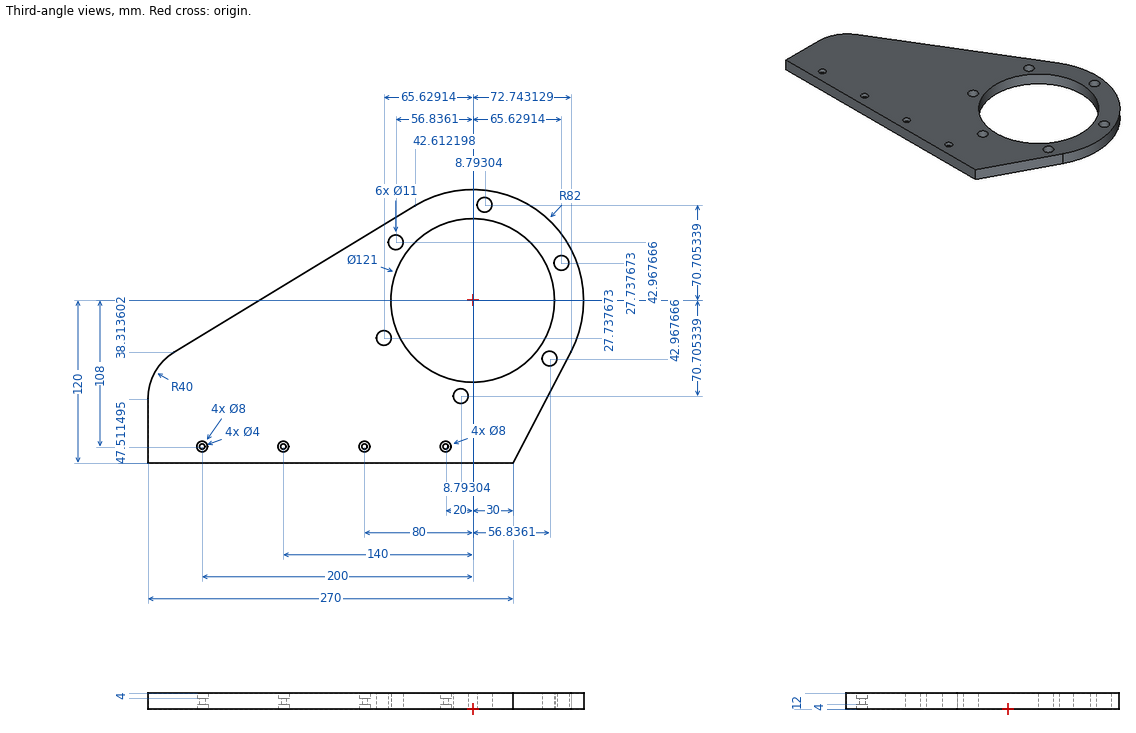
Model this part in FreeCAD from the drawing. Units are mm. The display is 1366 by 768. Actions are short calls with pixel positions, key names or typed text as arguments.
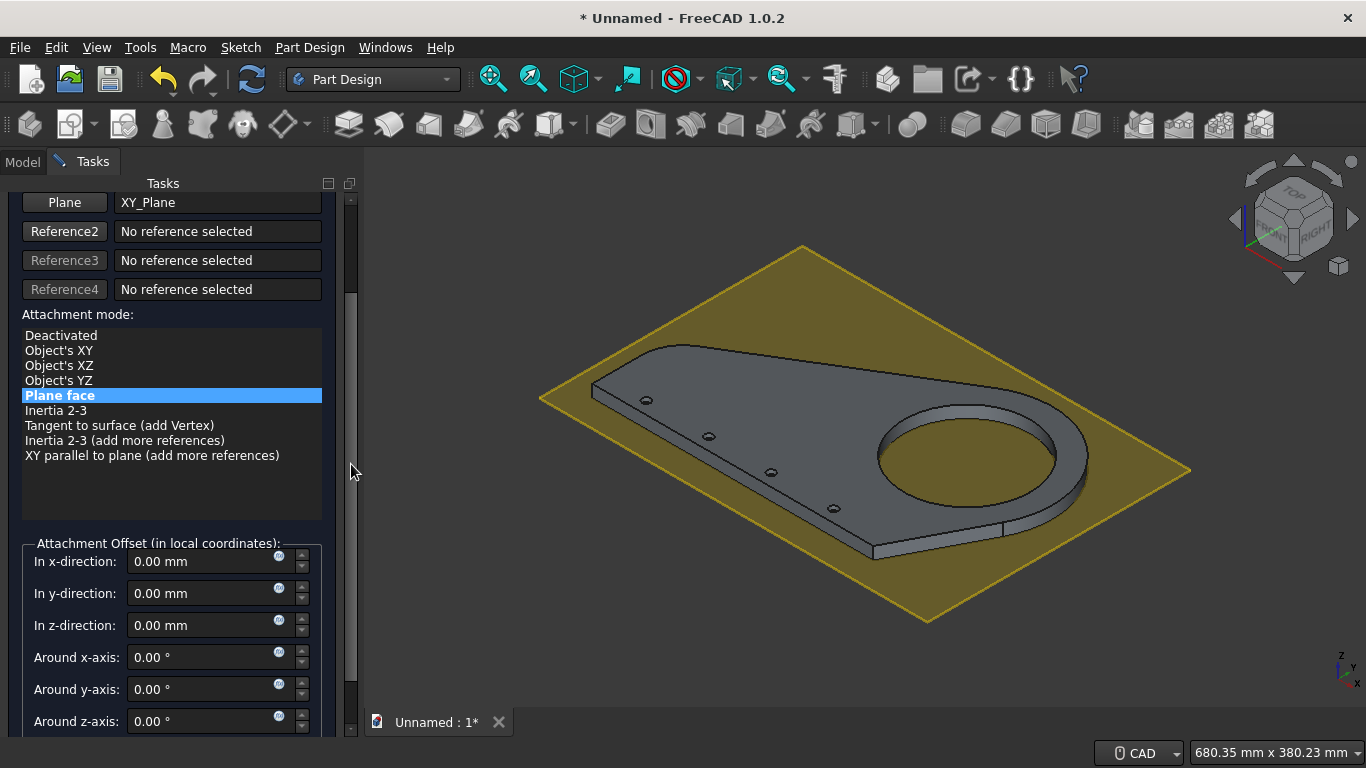
triple_click(210, 625)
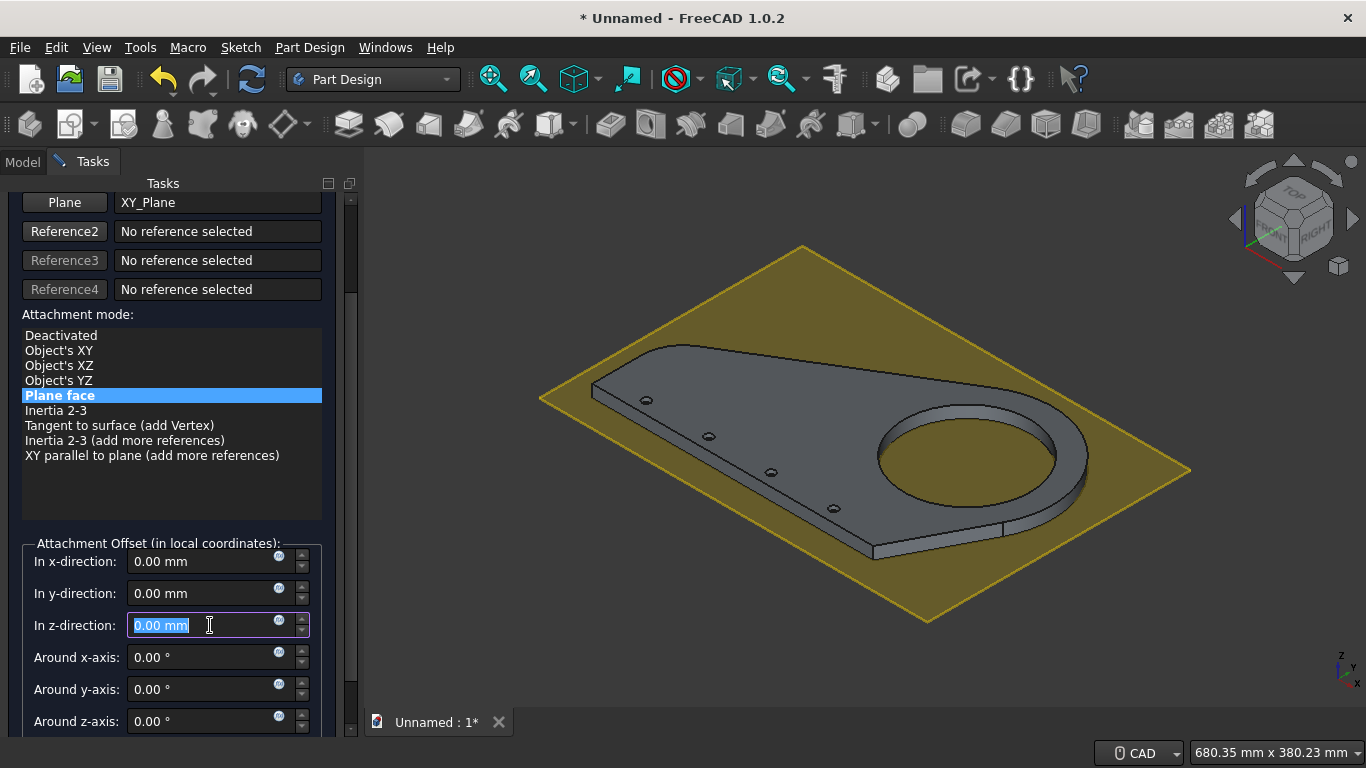
text(4)
key(Tab)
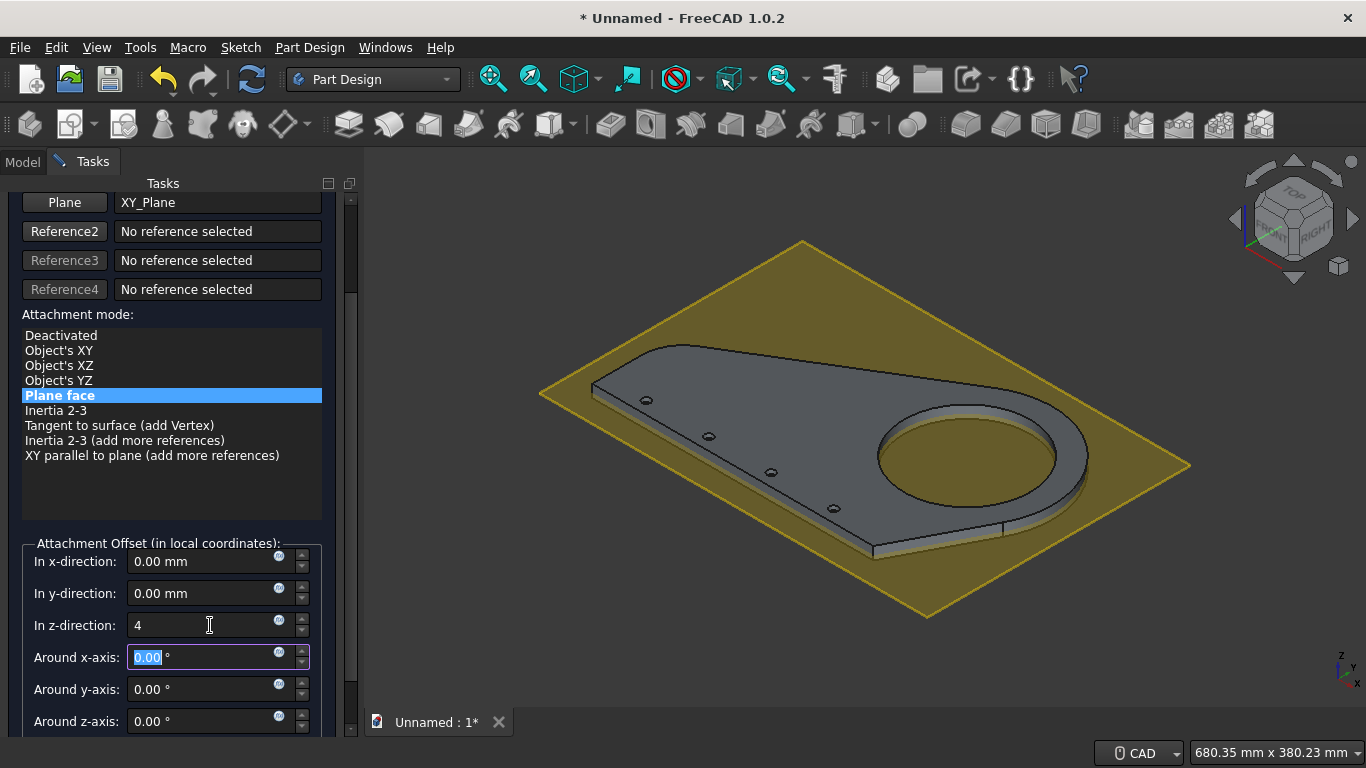
scroll(351, 464, up, 3)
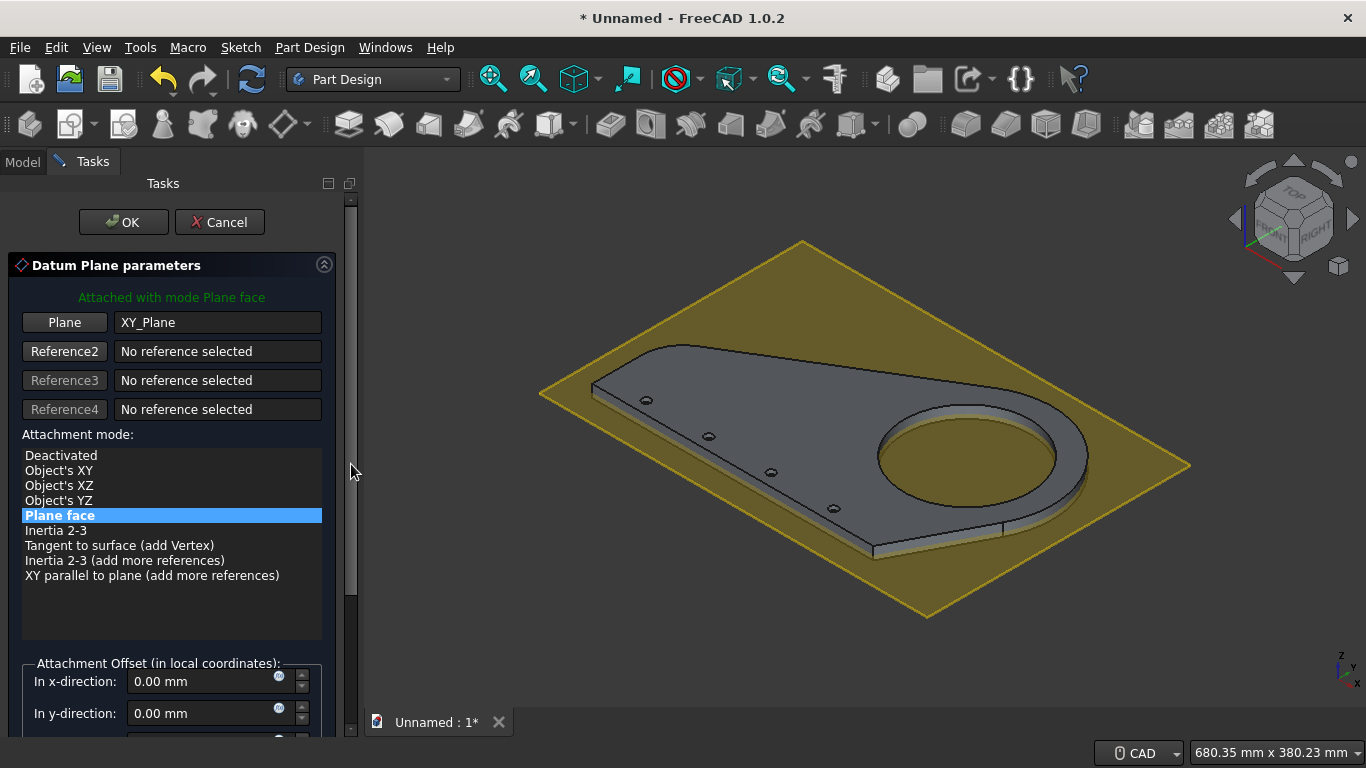
click(124, 222)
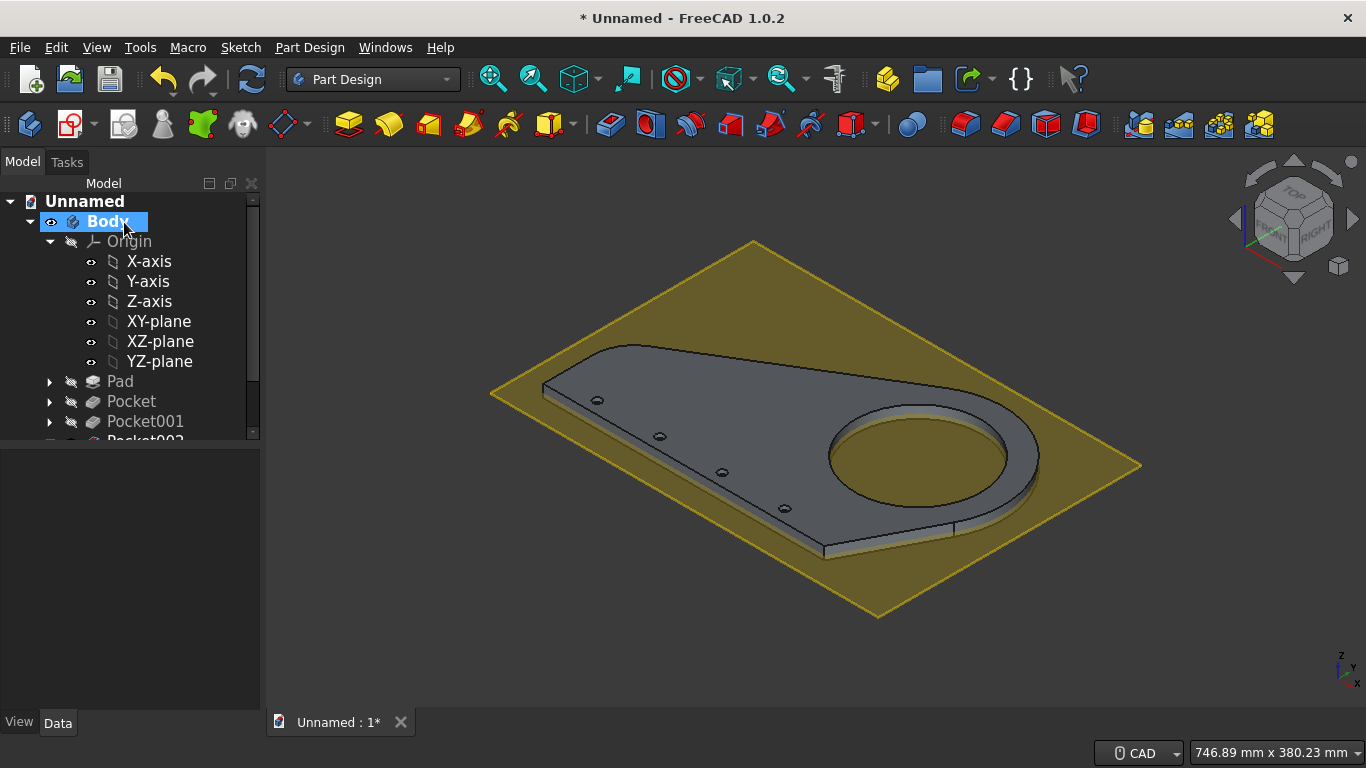
scroll(100, 317, down, 3)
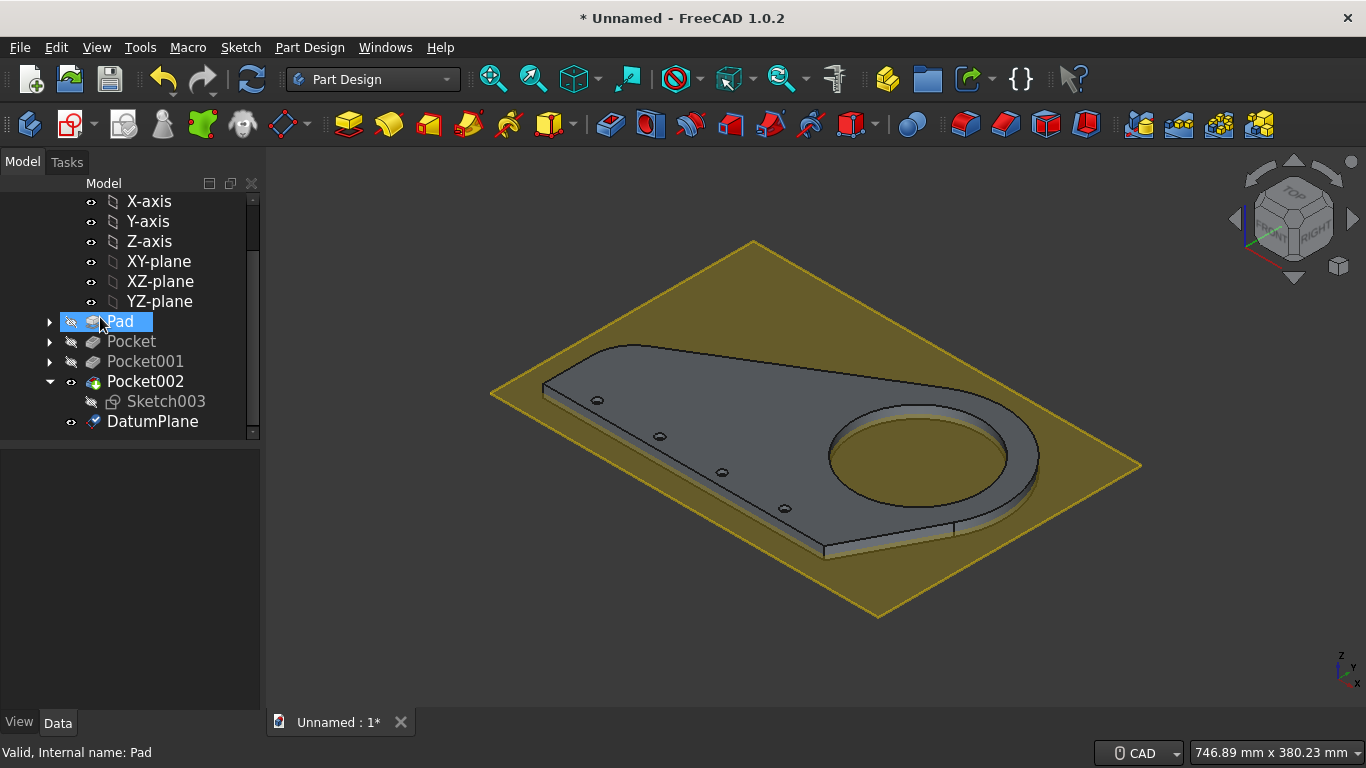
click(116, 422)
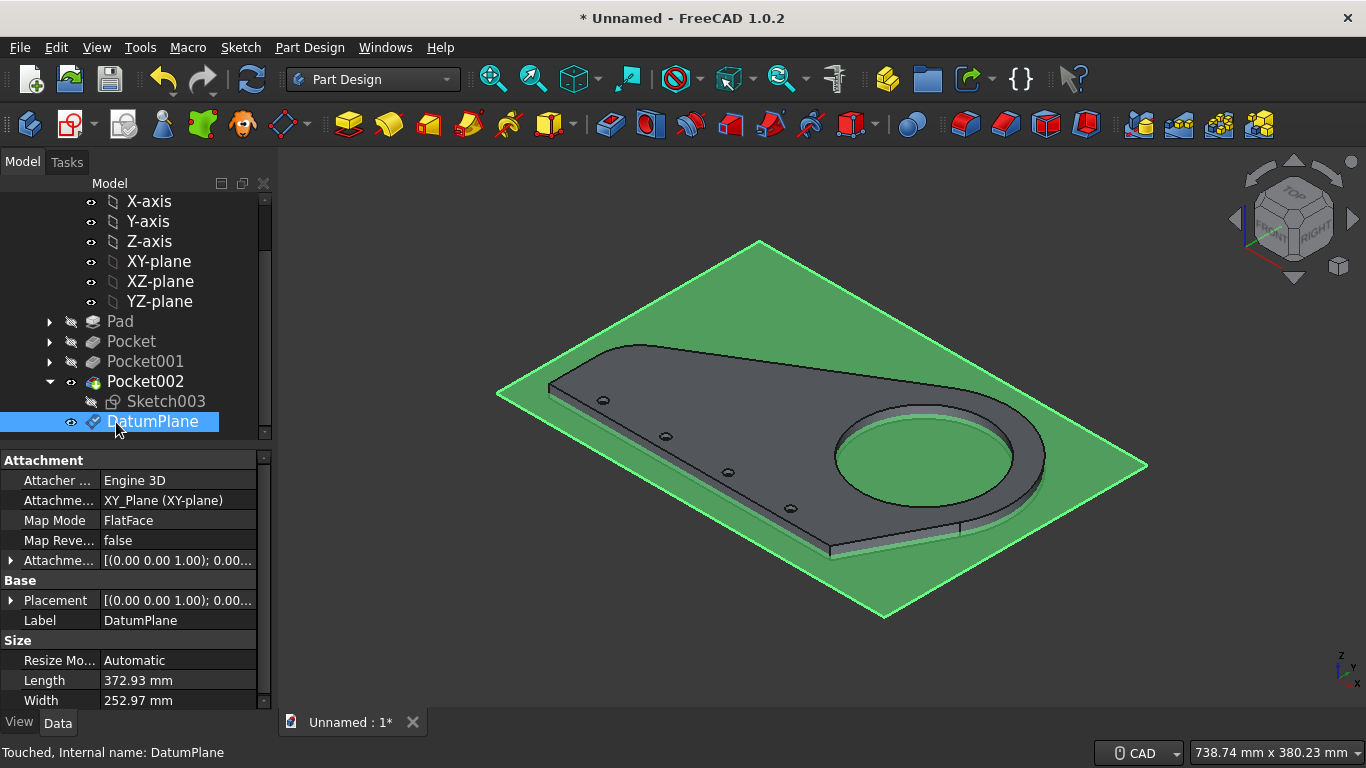
click(70, 124)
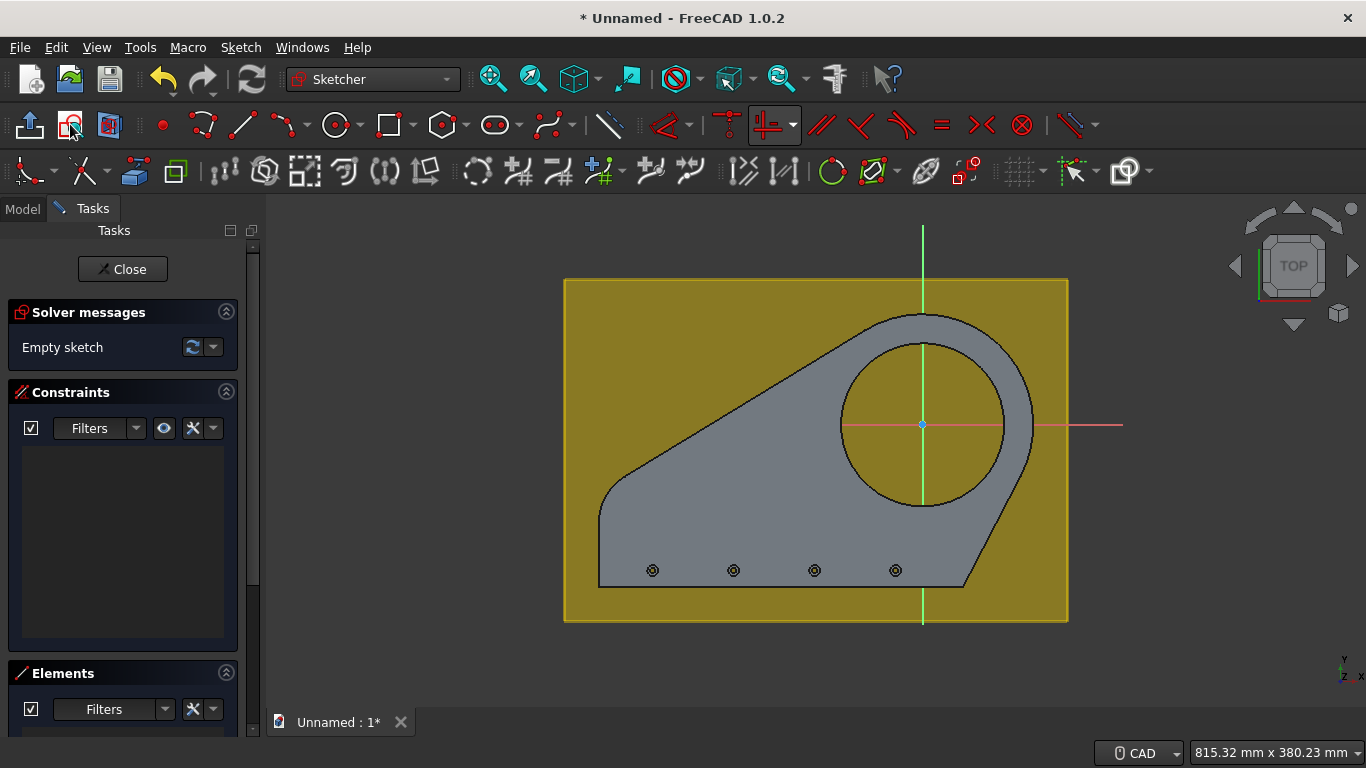
click(110, 126)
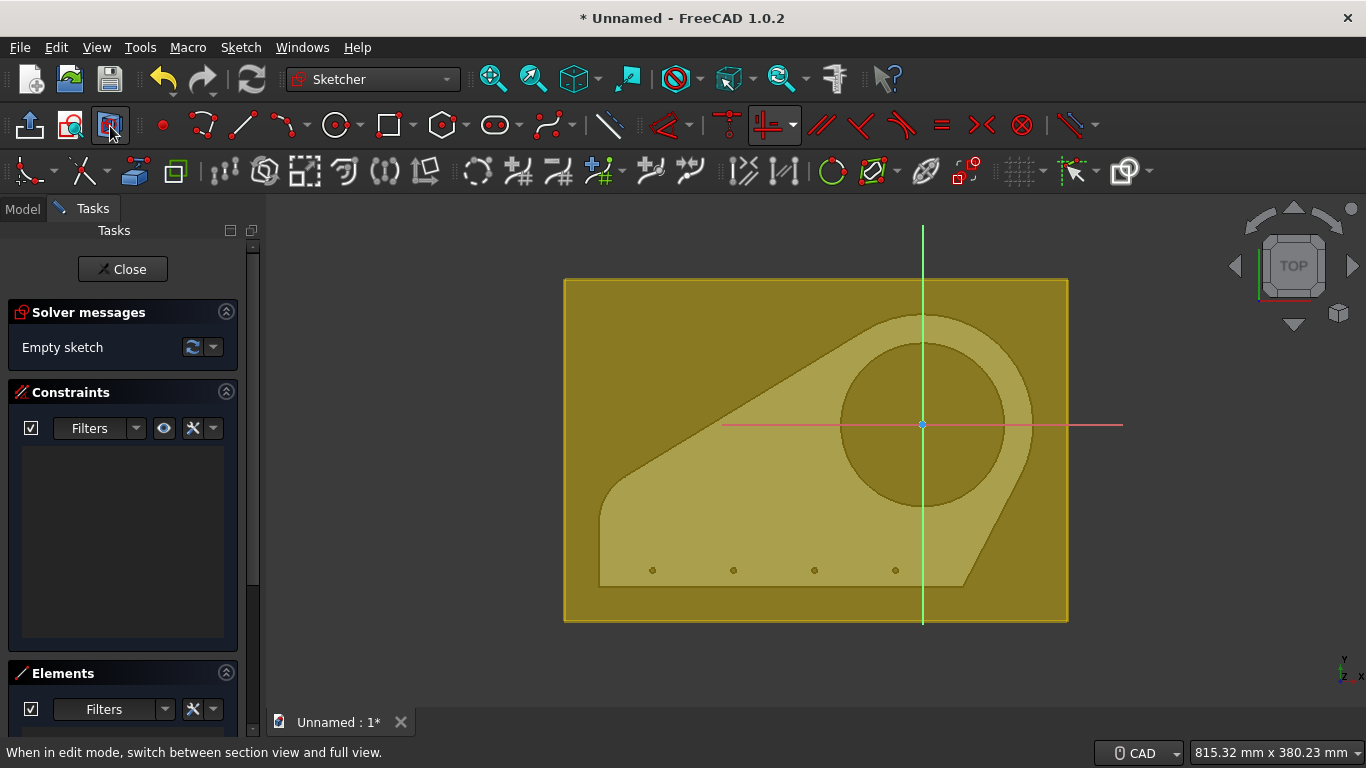
scroll(816, 541, up, 4)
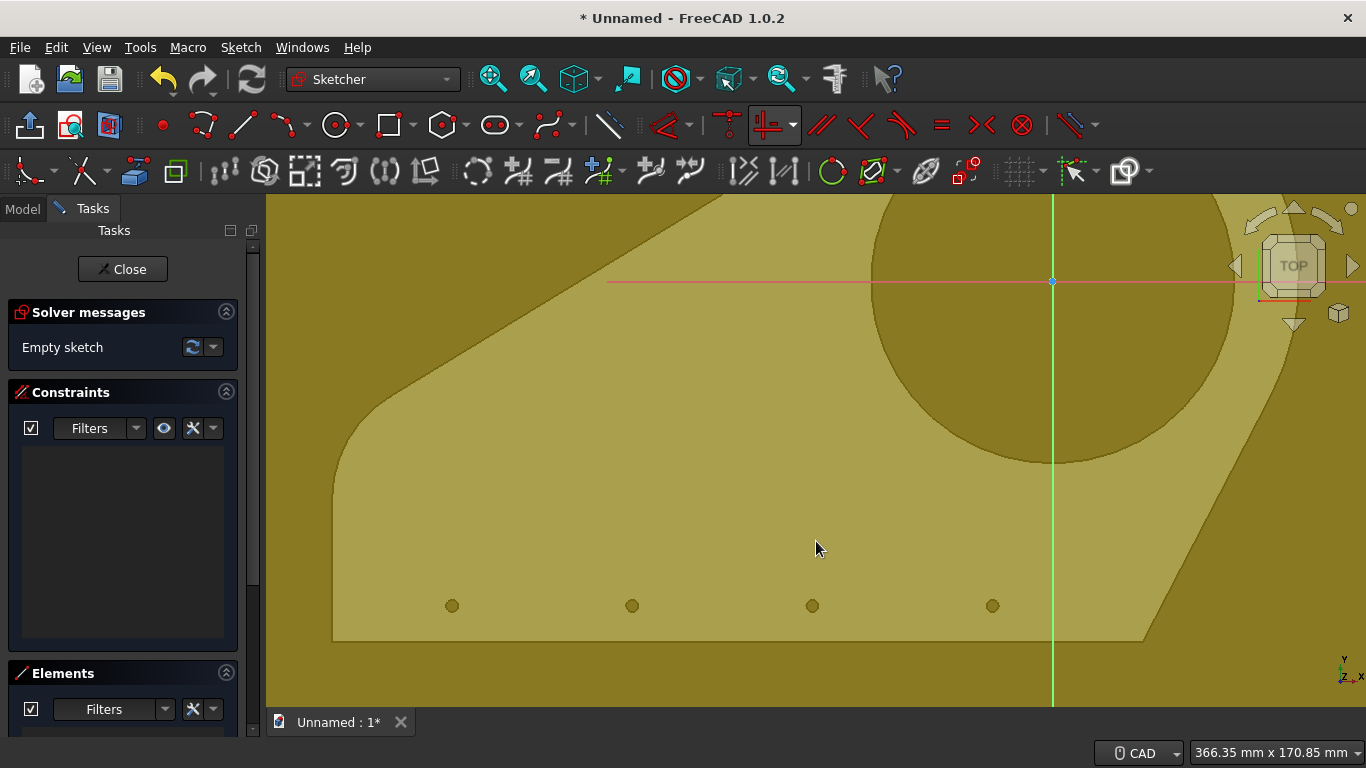
click(336, 126)